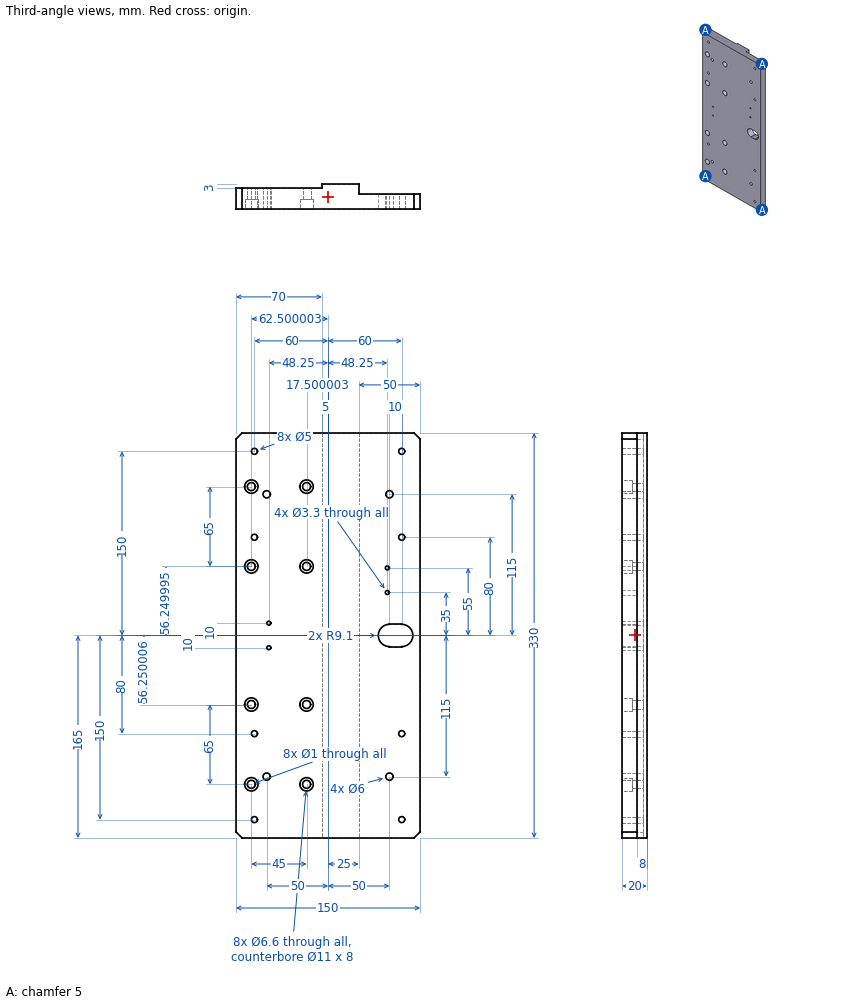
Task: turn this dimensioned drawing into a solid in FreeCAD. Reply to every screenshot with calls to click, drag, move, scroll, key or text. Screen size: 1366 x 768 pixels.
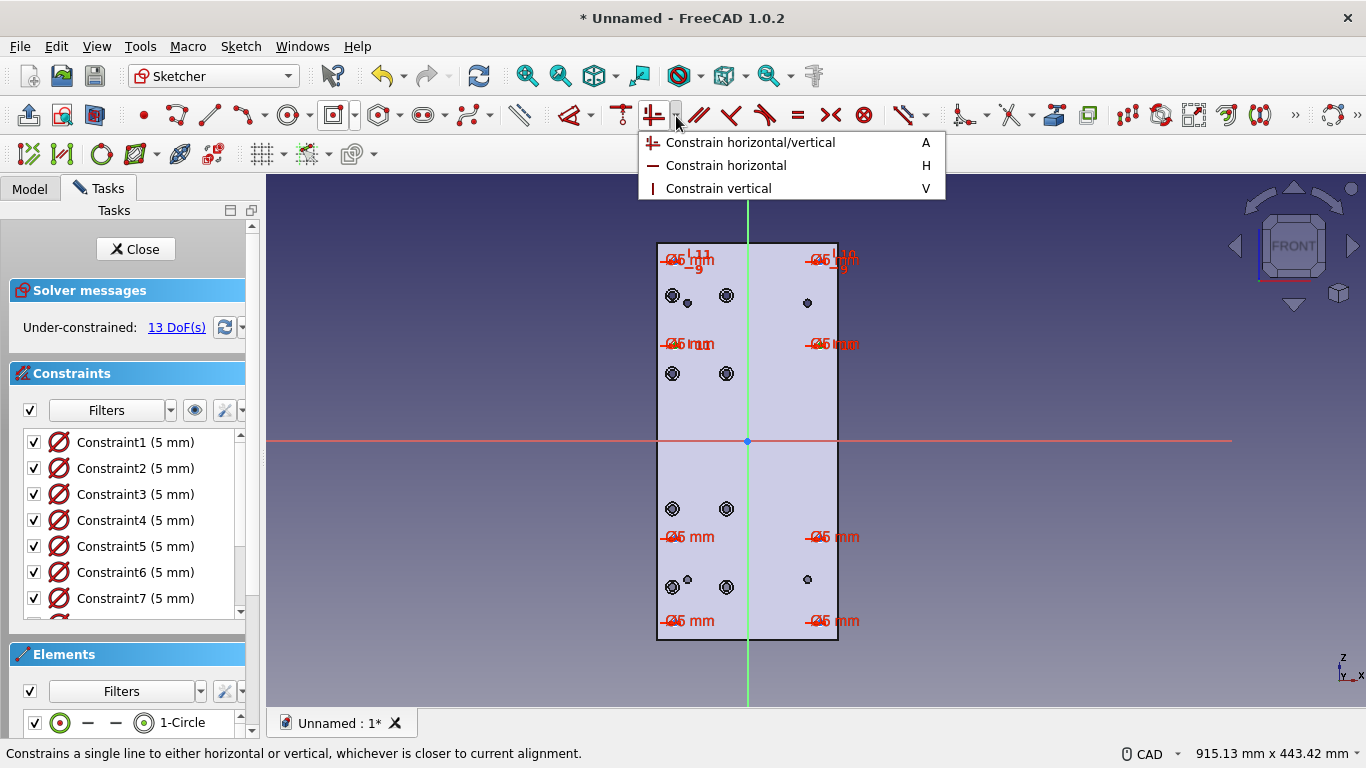
click(792, 166)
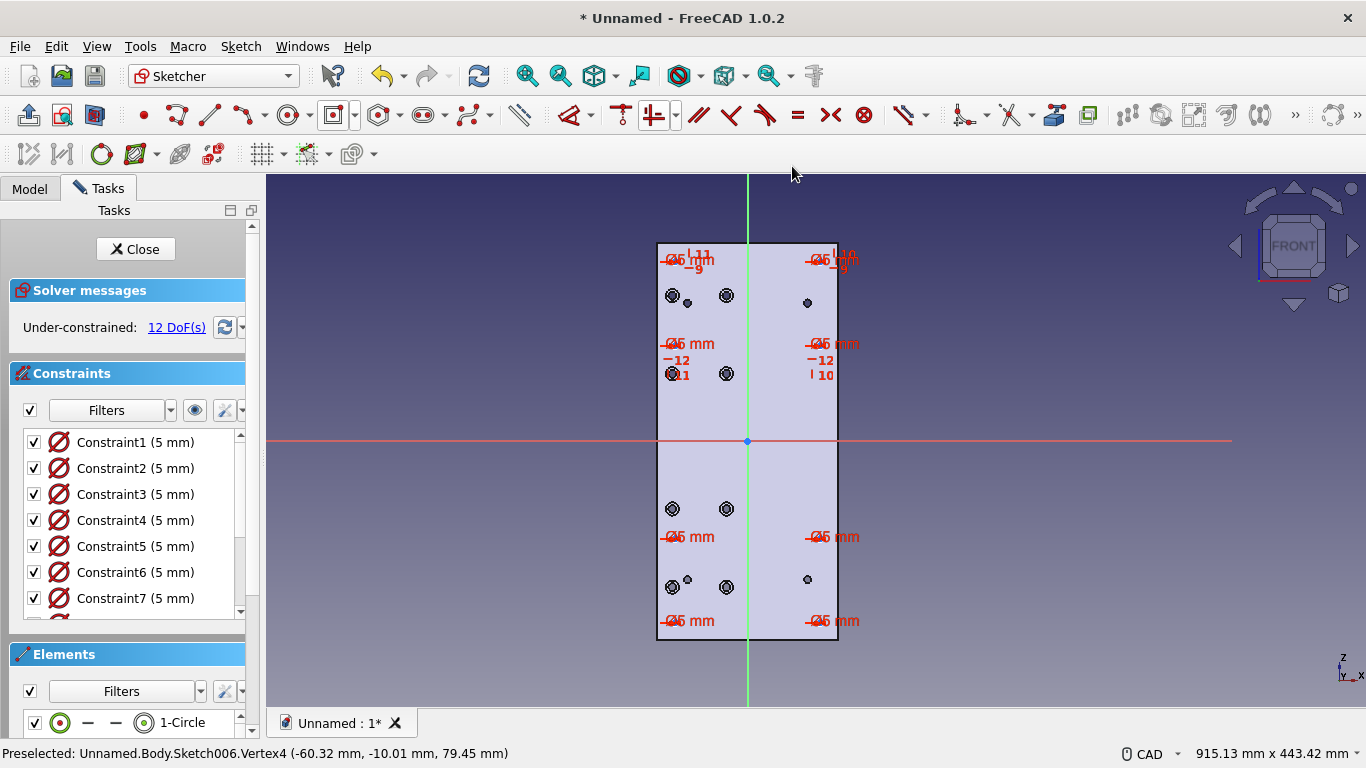
click(675, 346)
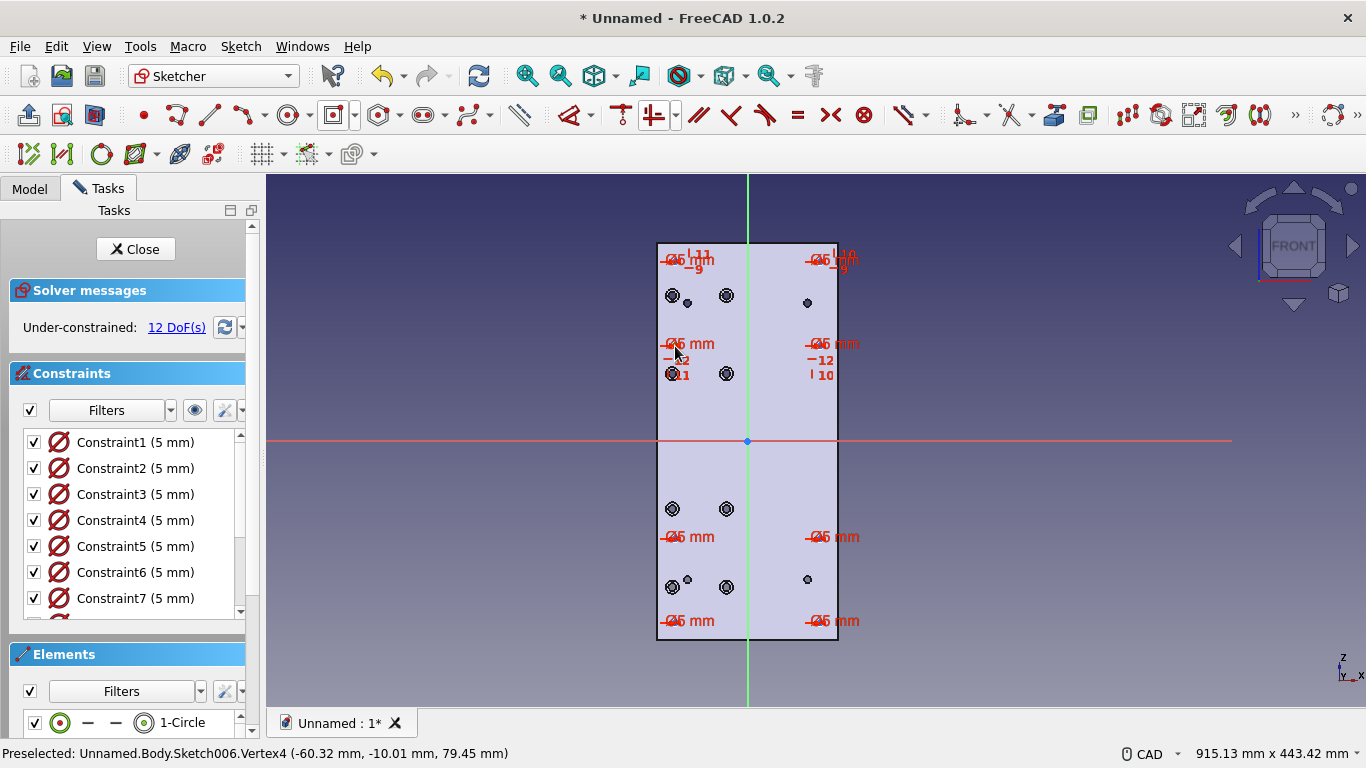
click(675, 539)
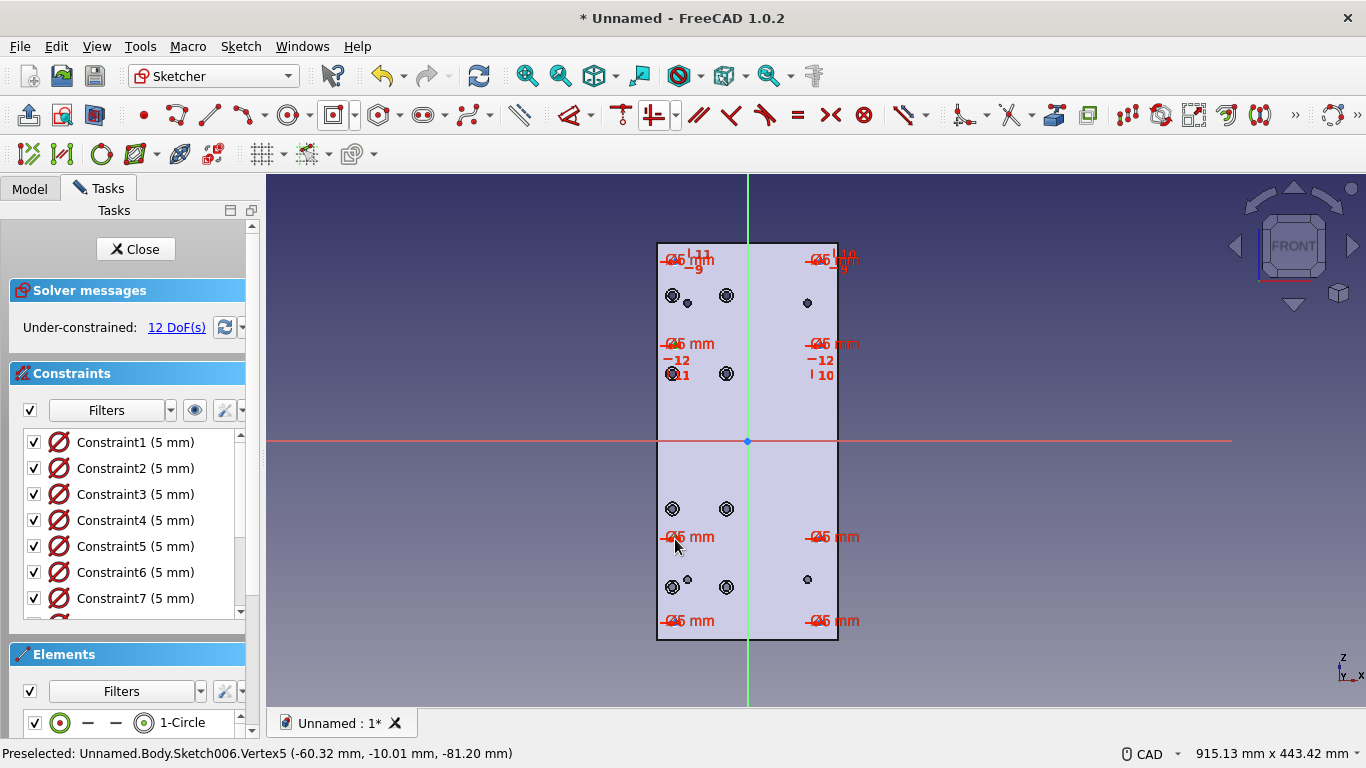
key(v)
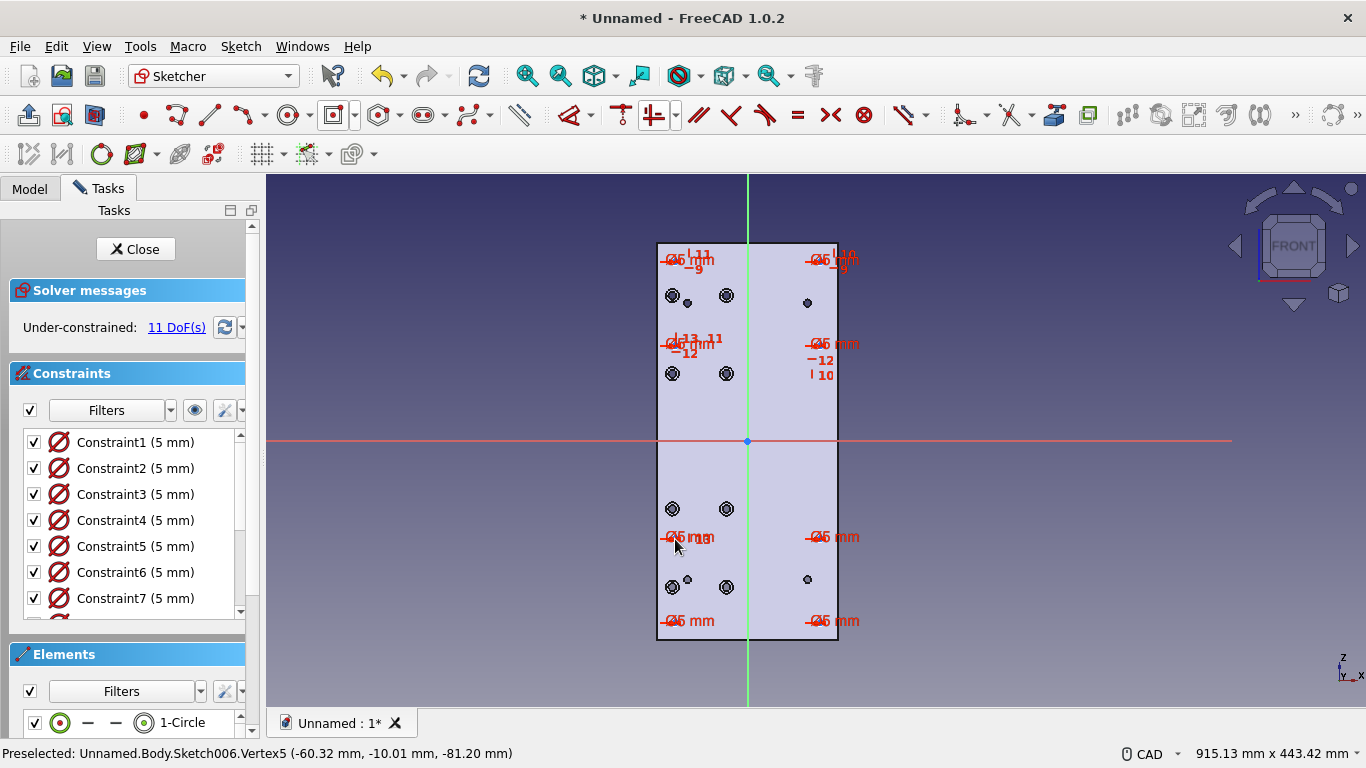
click(675, 539)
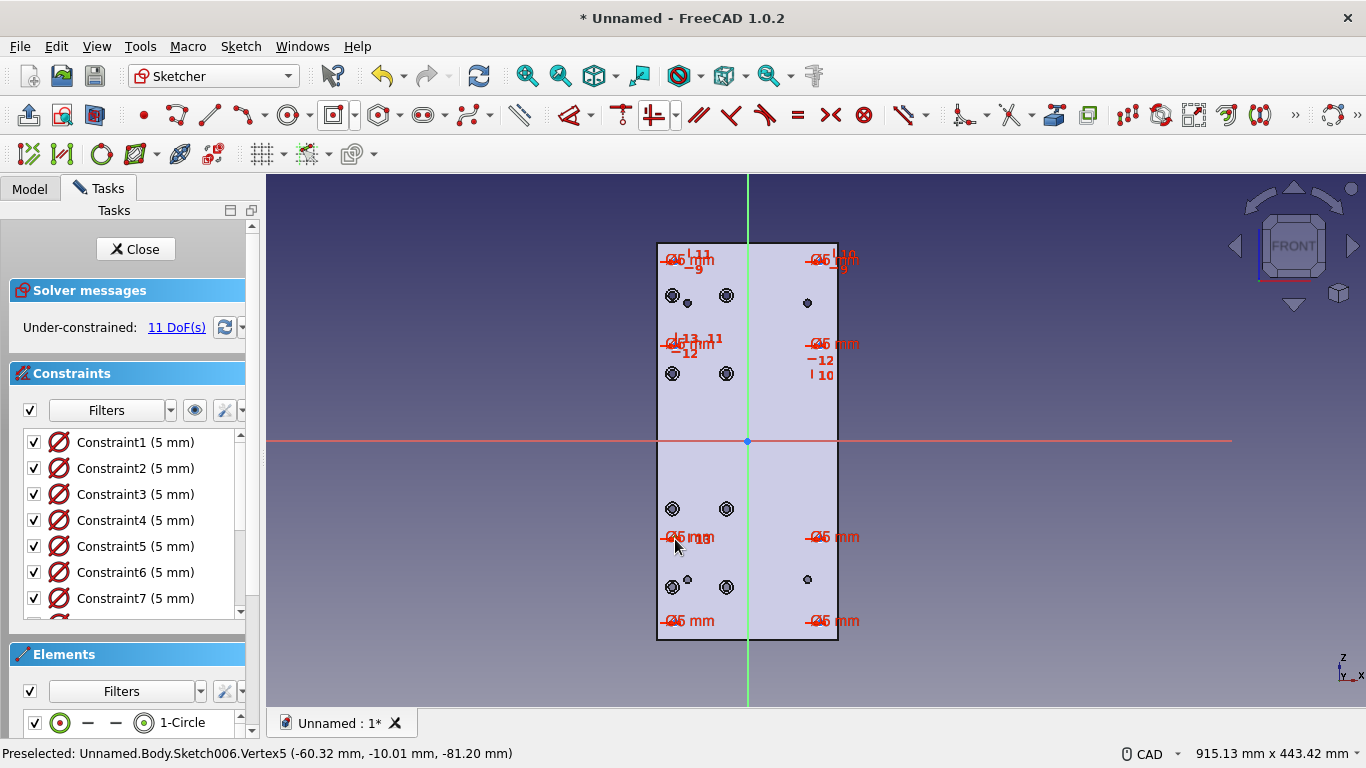
click(675, 623)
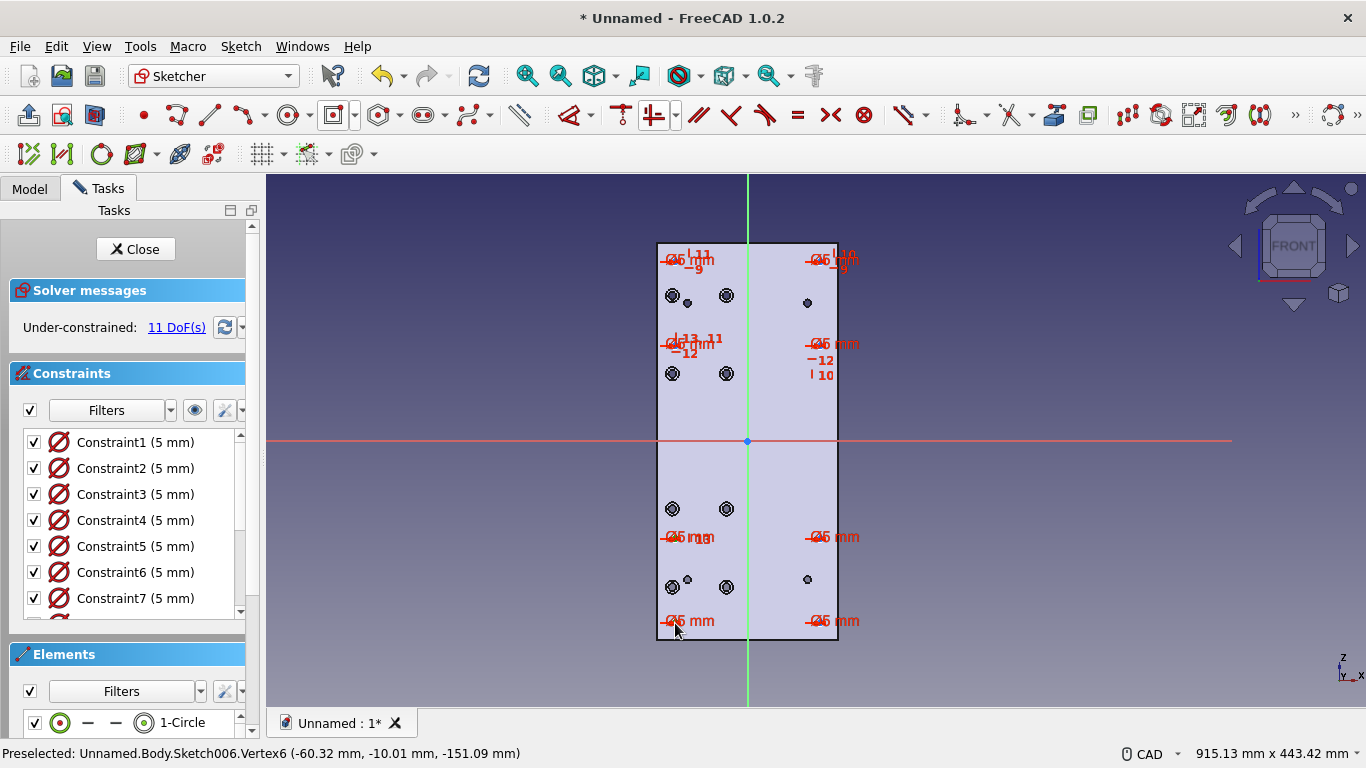
click(676, 116)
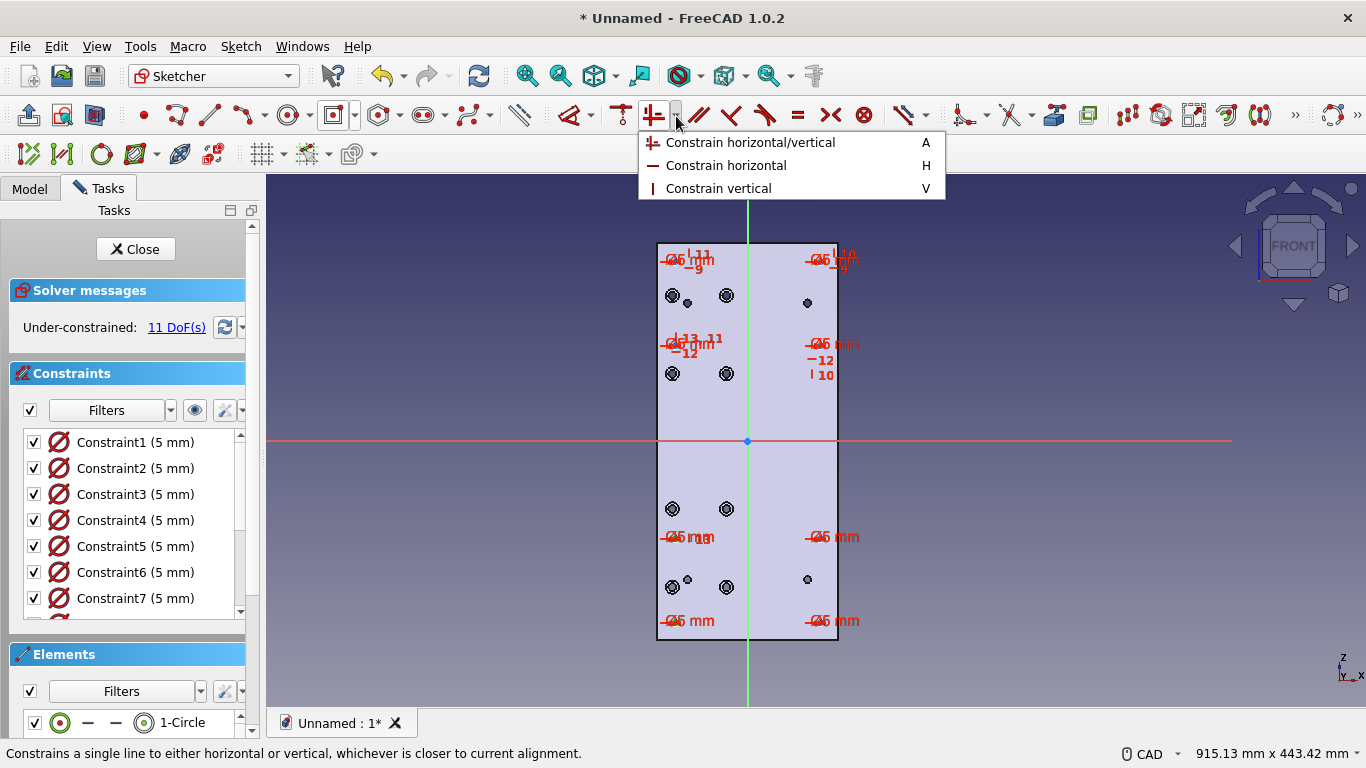
click(792, 188)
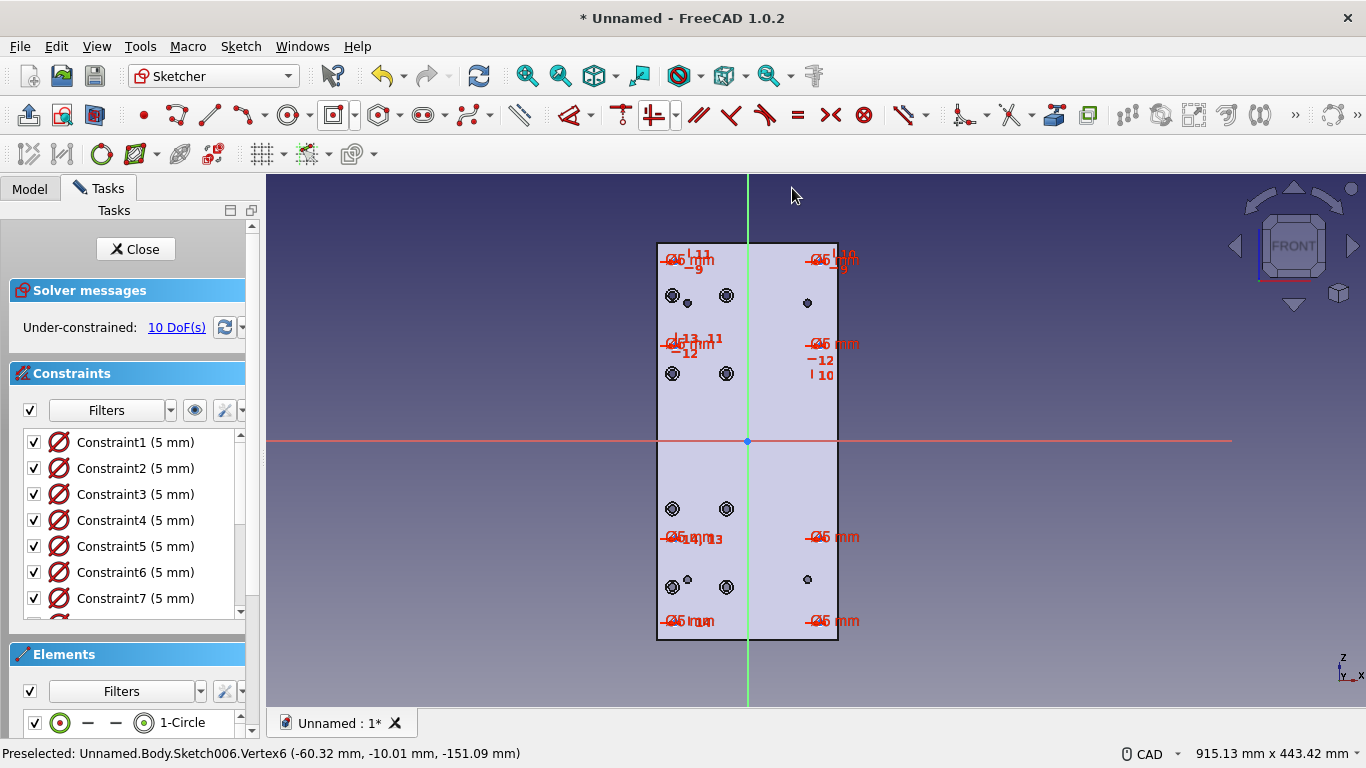
click(820, 346)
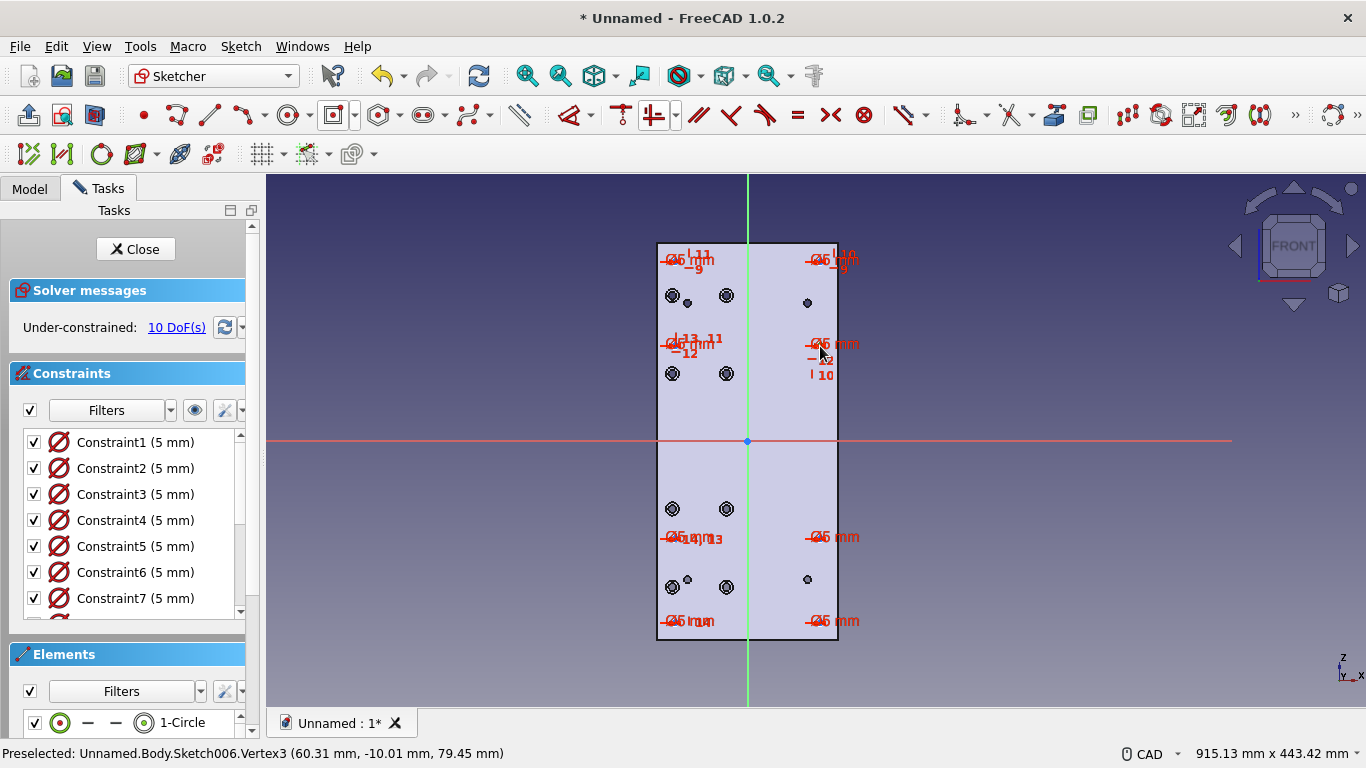
click(820, 623)